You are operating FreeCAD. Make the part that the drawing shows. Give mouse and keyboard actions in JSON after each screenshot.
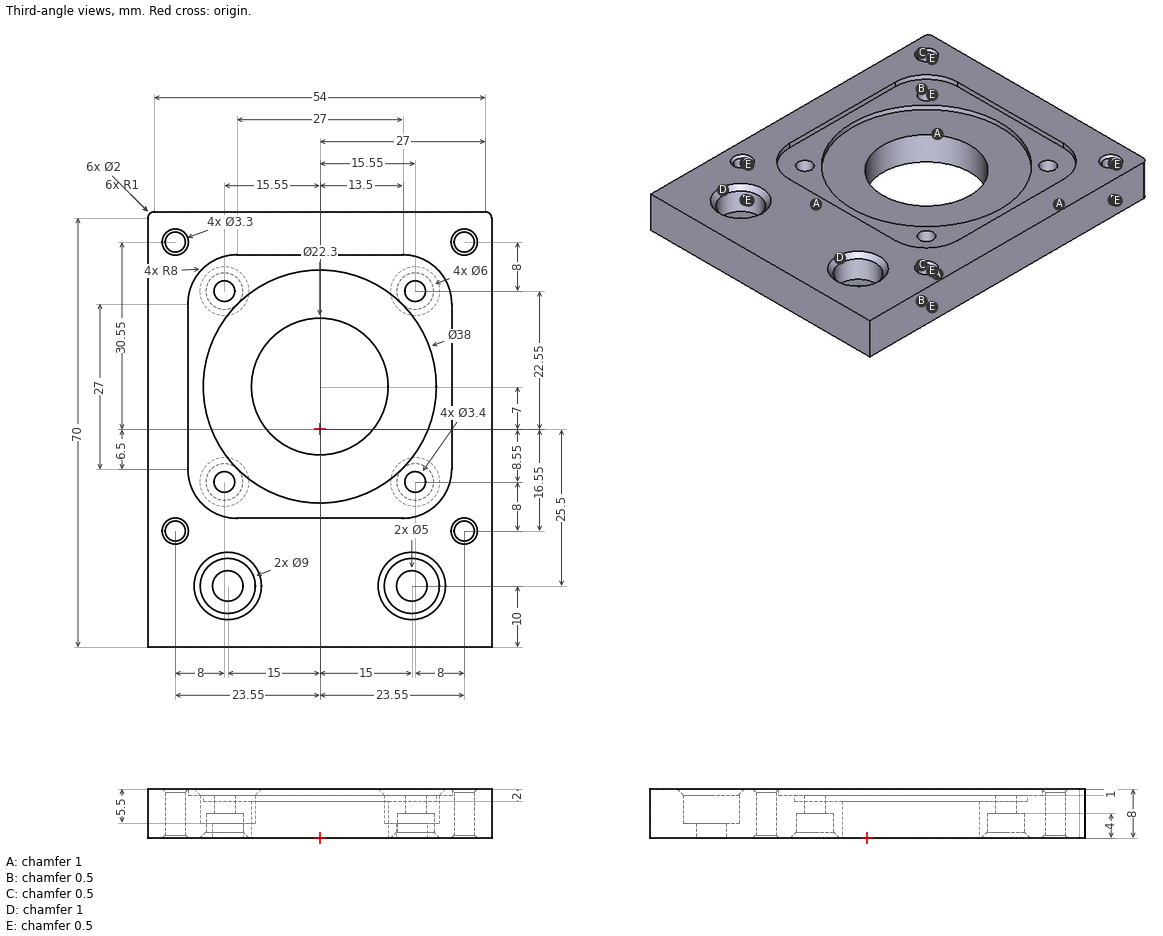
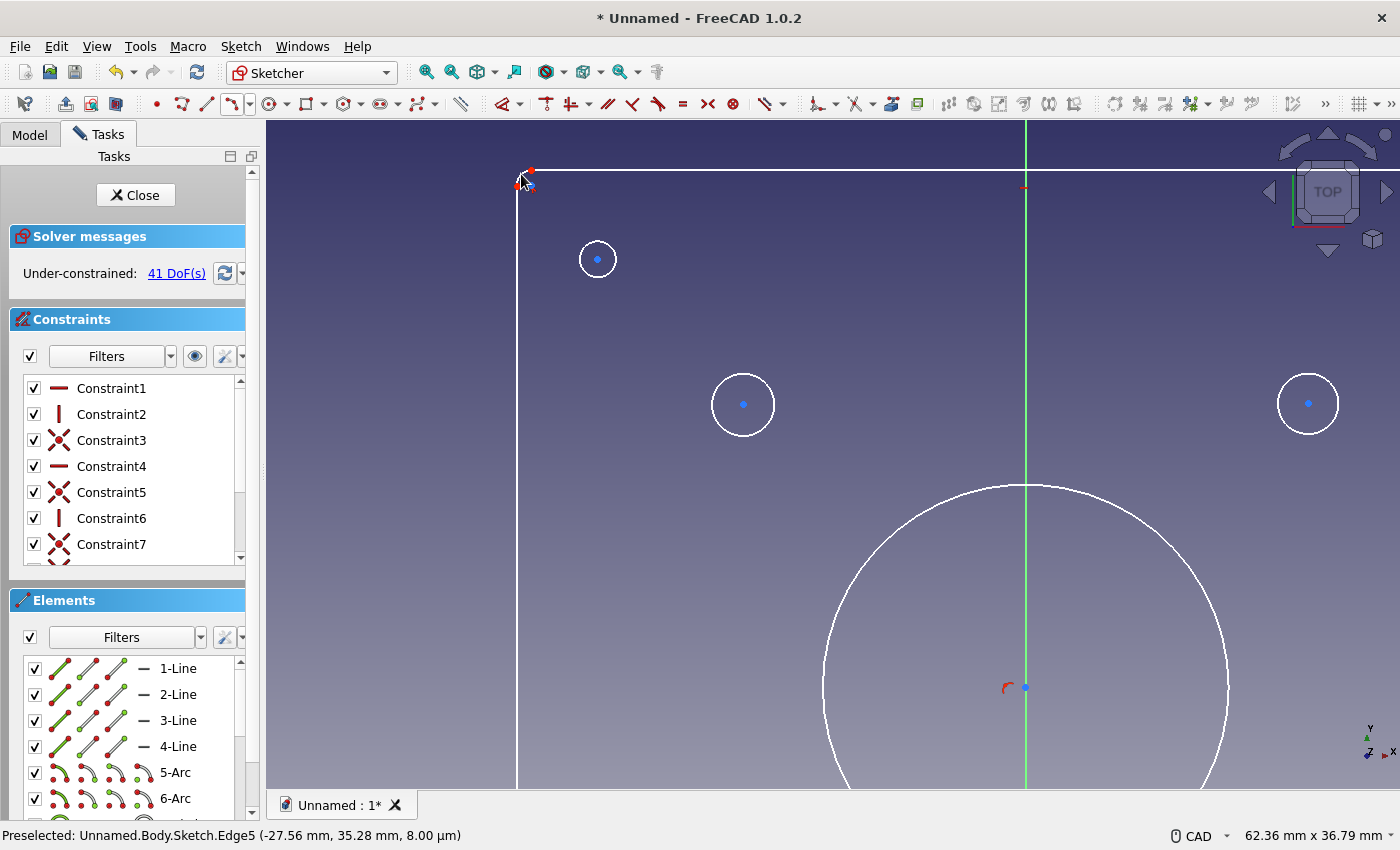
{"action": "left_click", "coordinate": [1222, 170]}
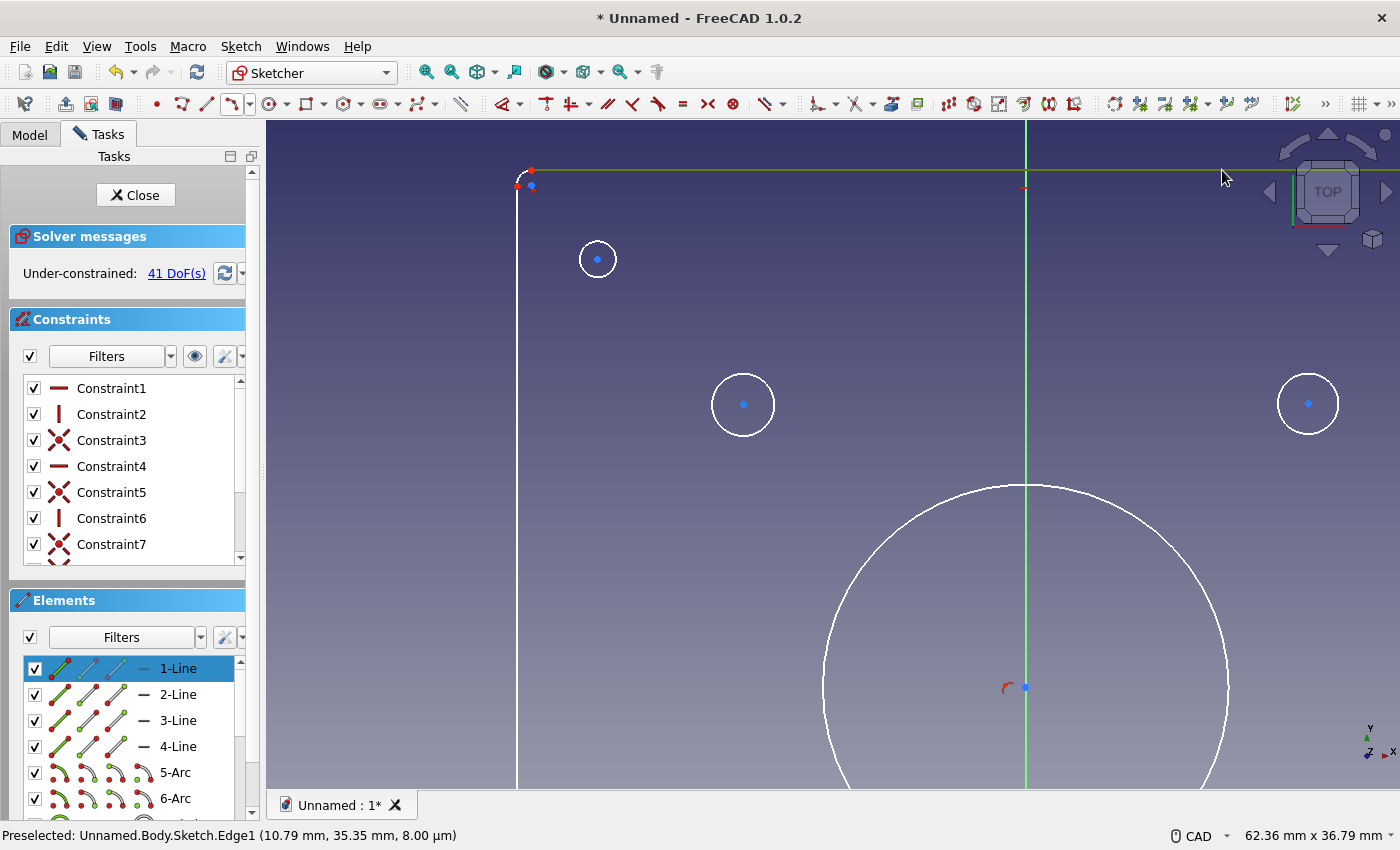
{"action": "scroll", "coordinate": [612, 246], "scroll_direction": "down", "scroll_amount": 5}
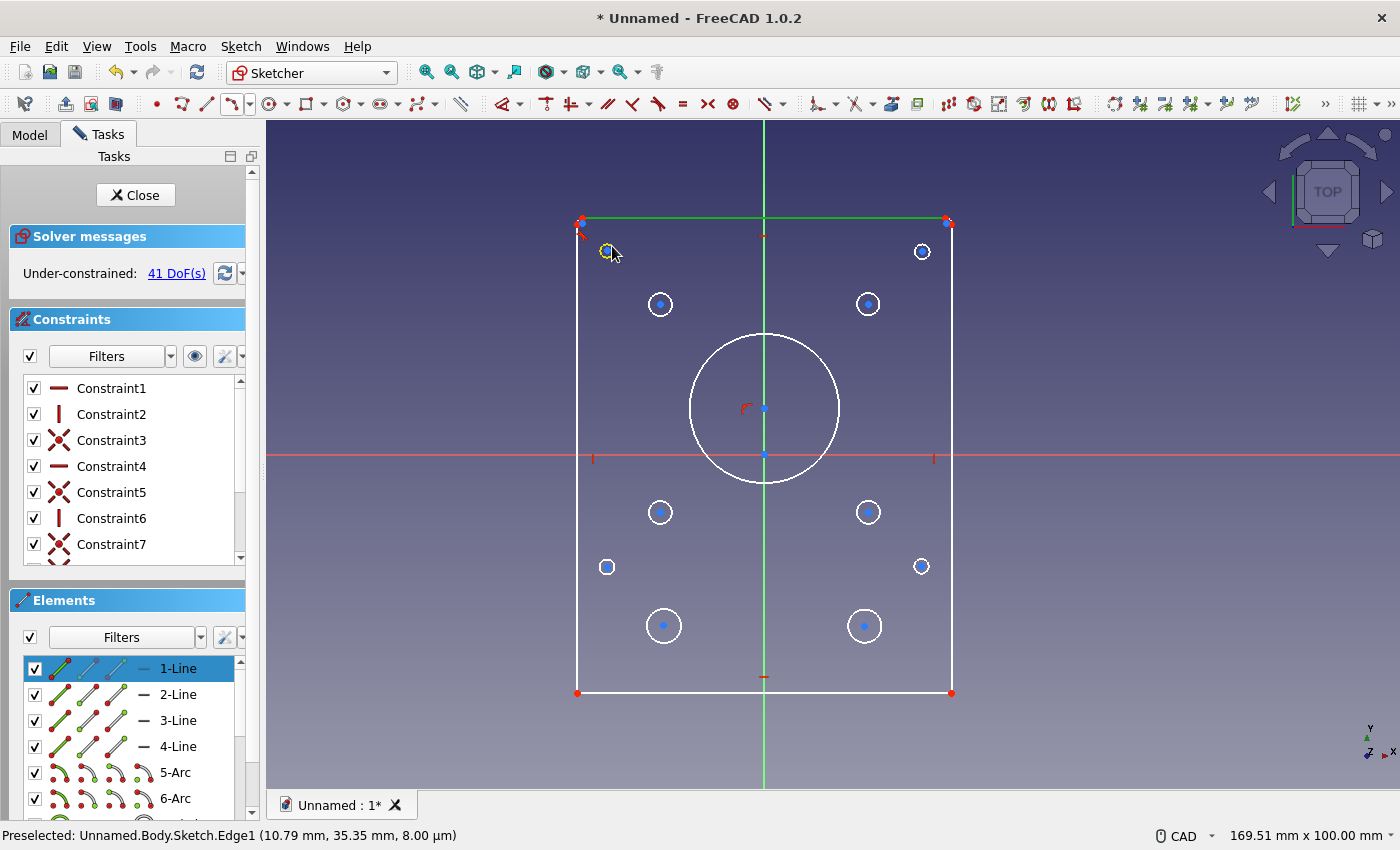
{"action": "scroll", "coordinate": [950, 220], "scroll_direction": "up", "scroll_amount": 6}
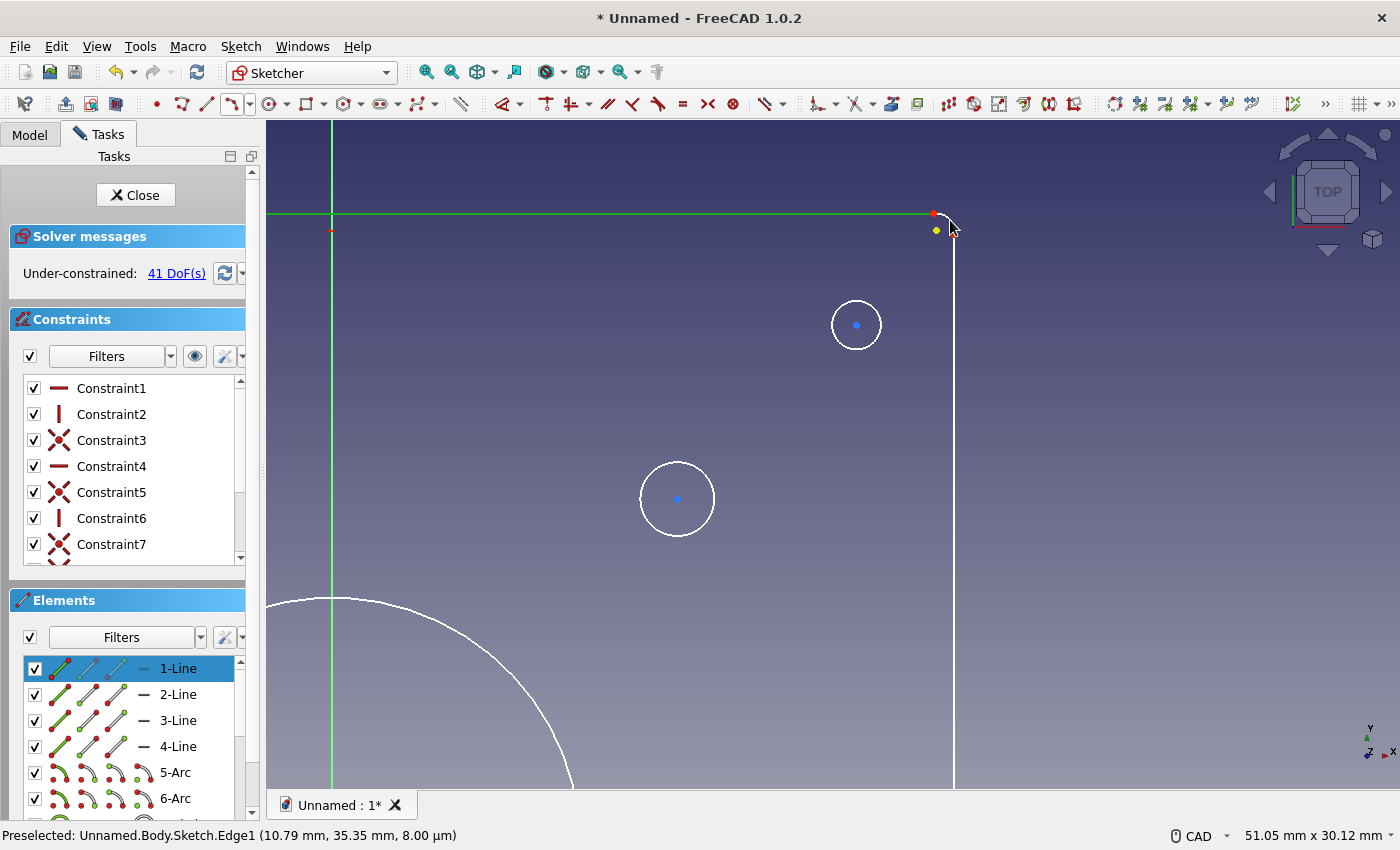
{"action": "left_click", "coordinate": [949, 219]}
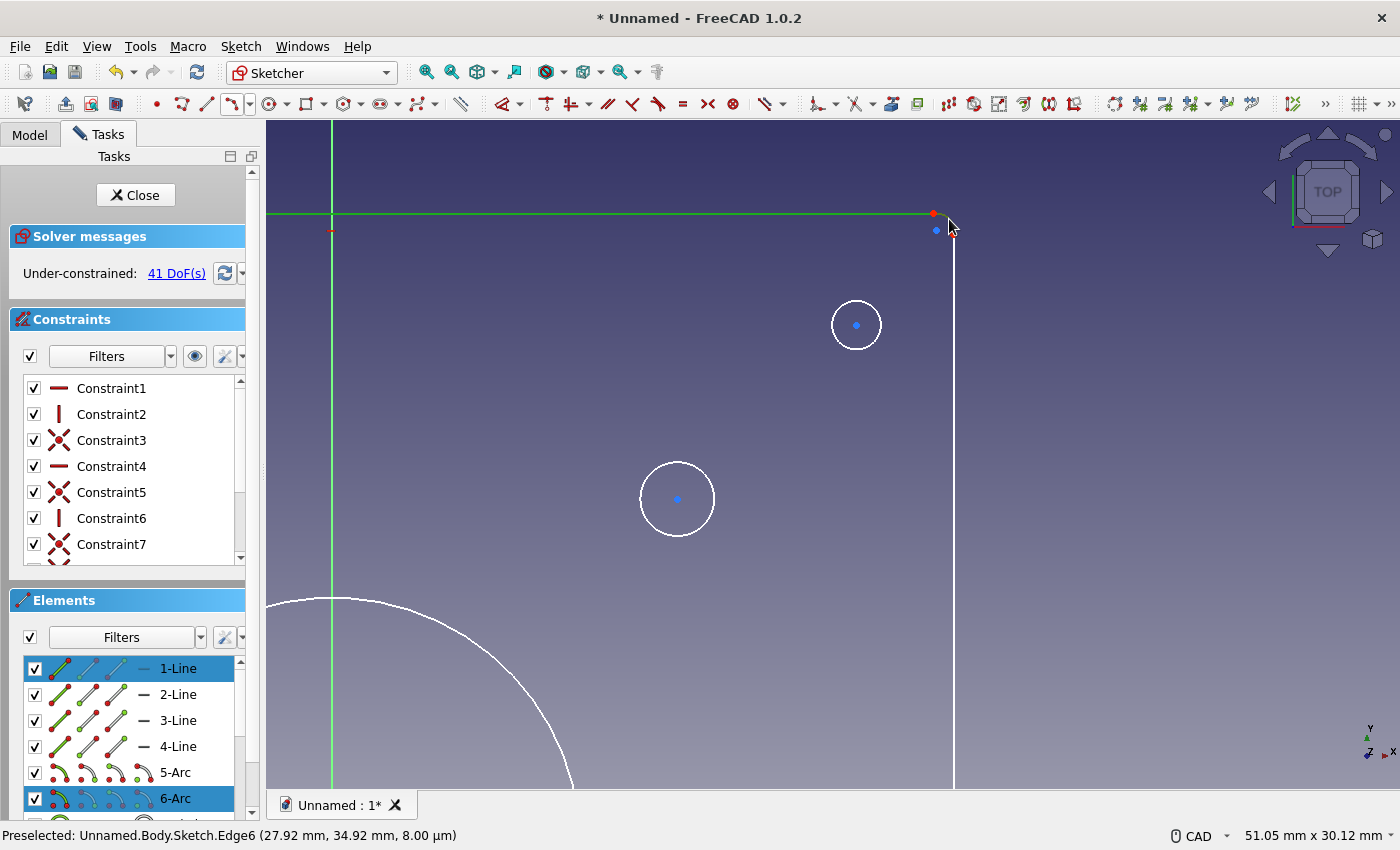
{"action": "left_click", "coordinate": [658, 104]}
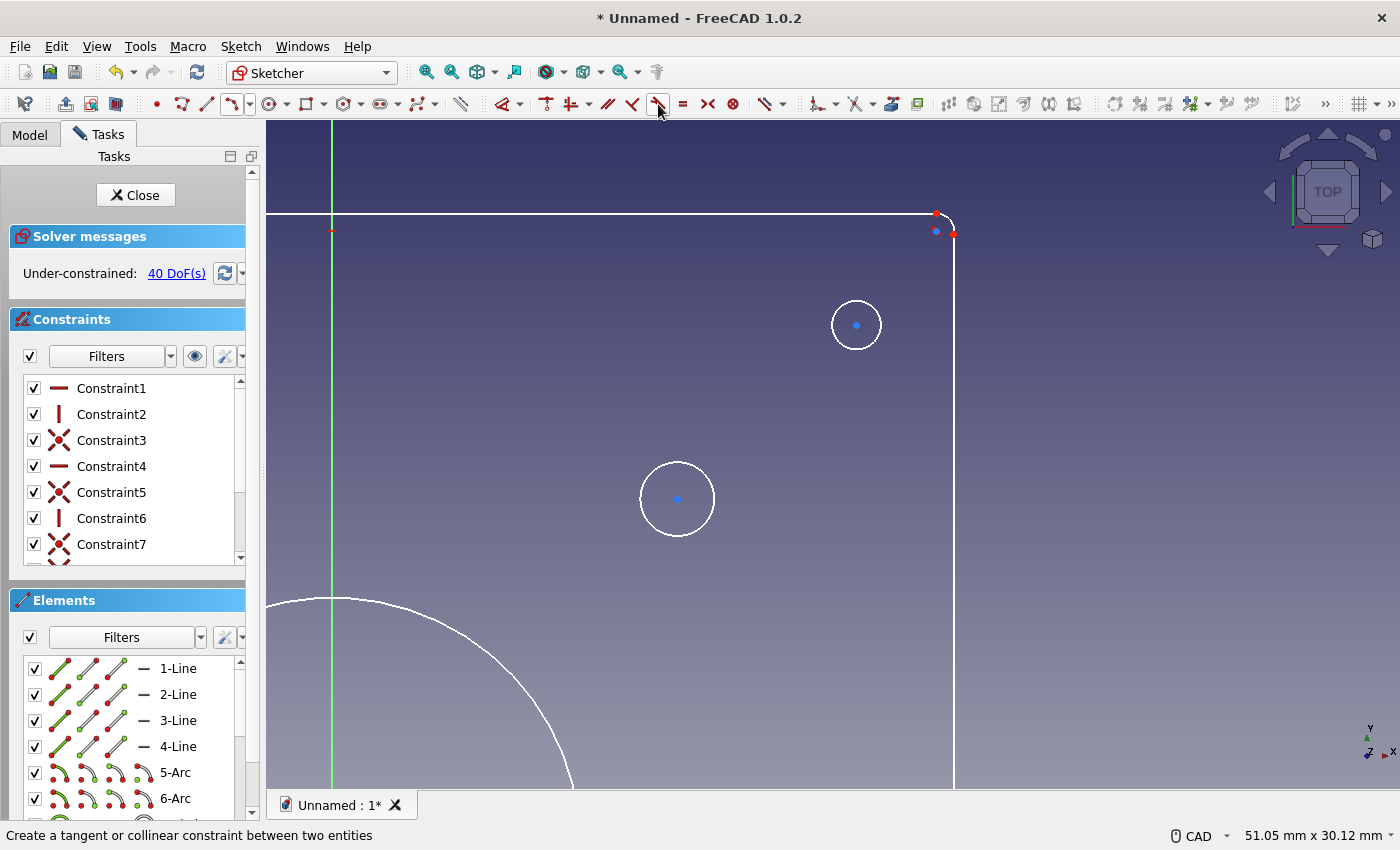
{"action": "scroll", "coordinate": [951, 220], "scroll_direction": "down", "scroll_amount": 6}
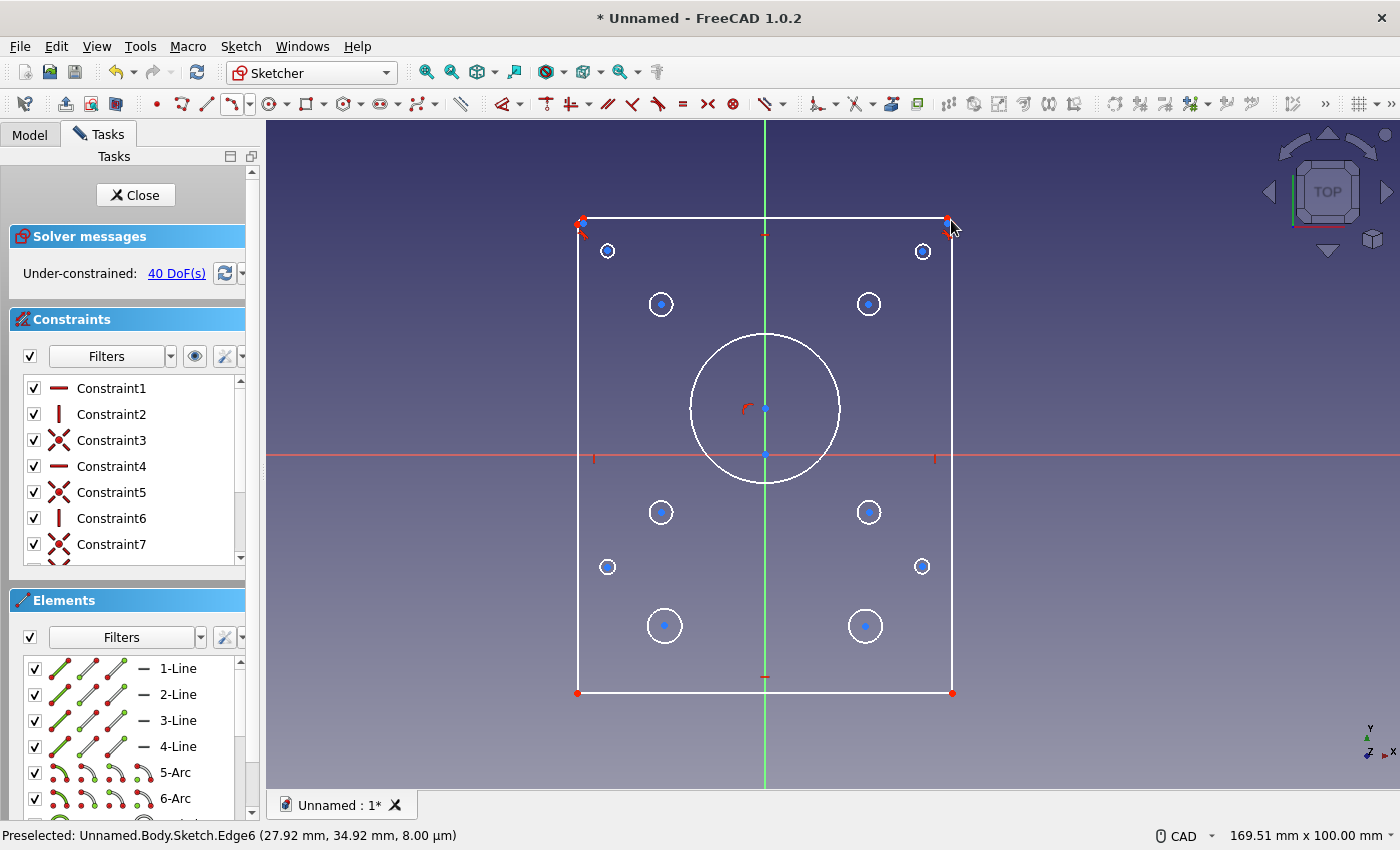
{"action": "left_click", "coordinate": [578, 365]}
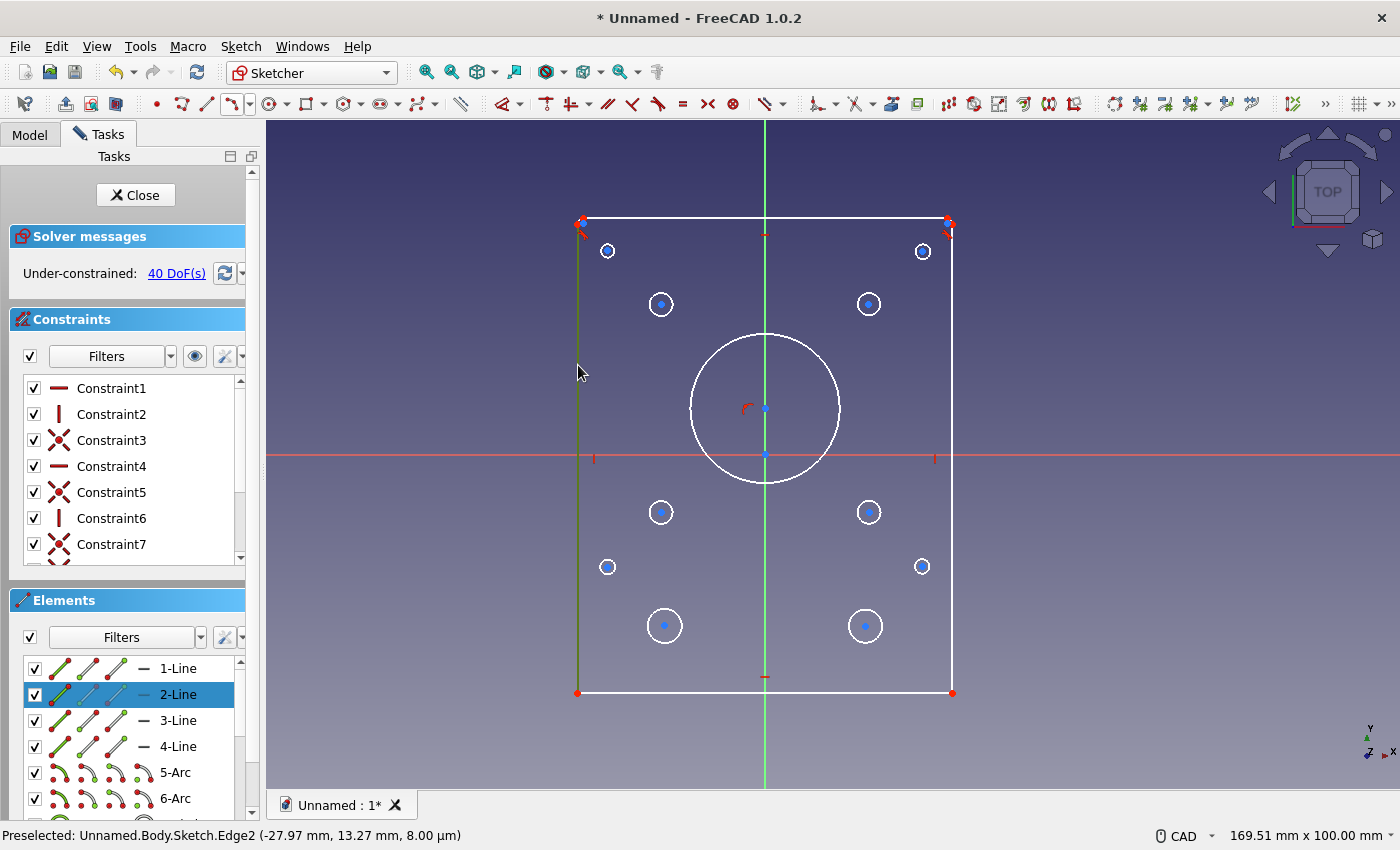
{"action": "scroll", "coordinate": [579, 220], "scroll_direction": "up", "scroll_amount": 6}